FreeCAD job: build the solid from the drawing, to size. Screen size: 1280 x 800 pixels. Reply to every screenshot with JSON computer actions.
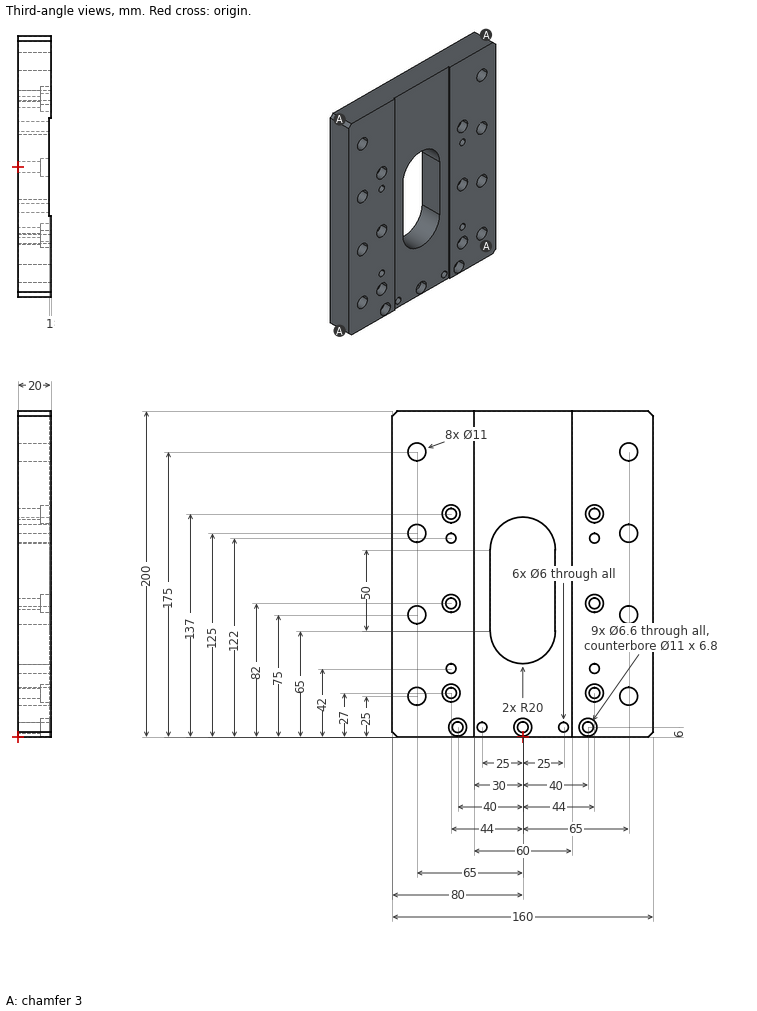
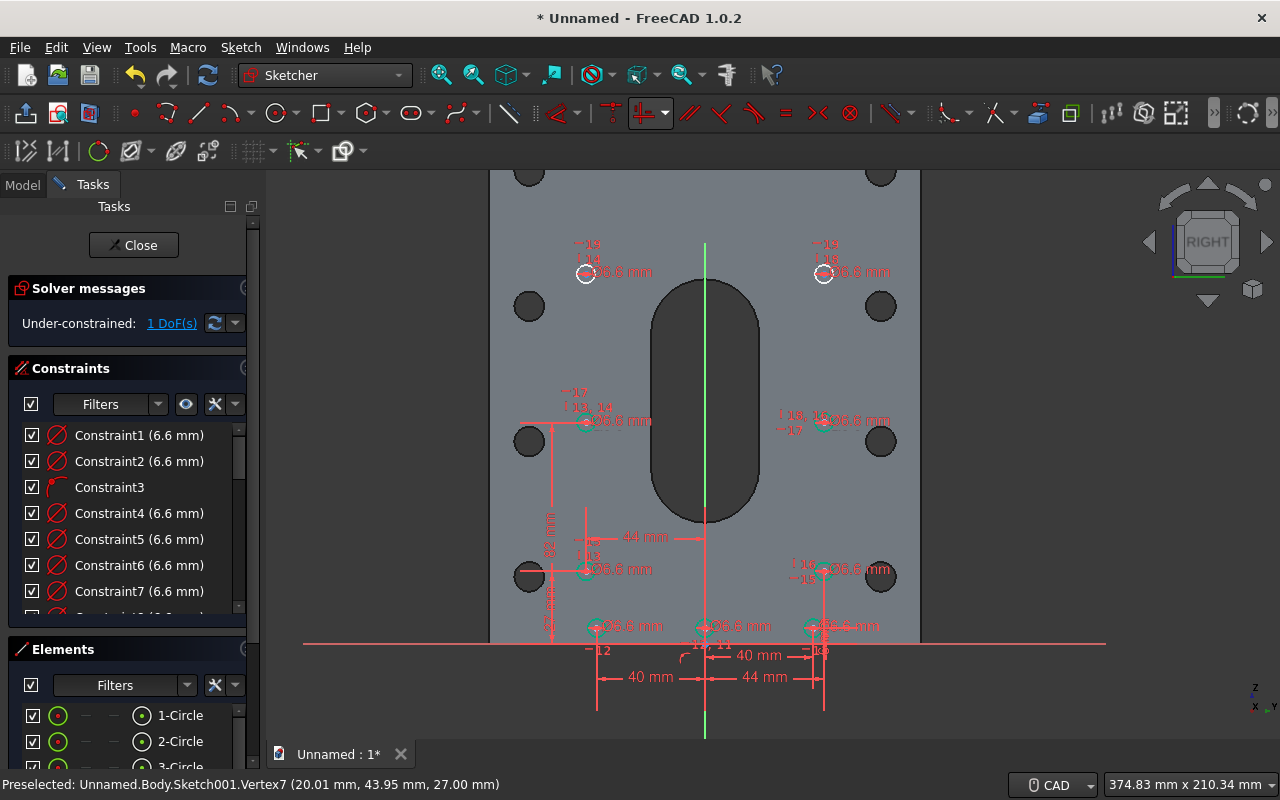
{"action": "left_click", "coordinate": [586, 274]}
{"action": "left_click", "coordinate": [552, 459]}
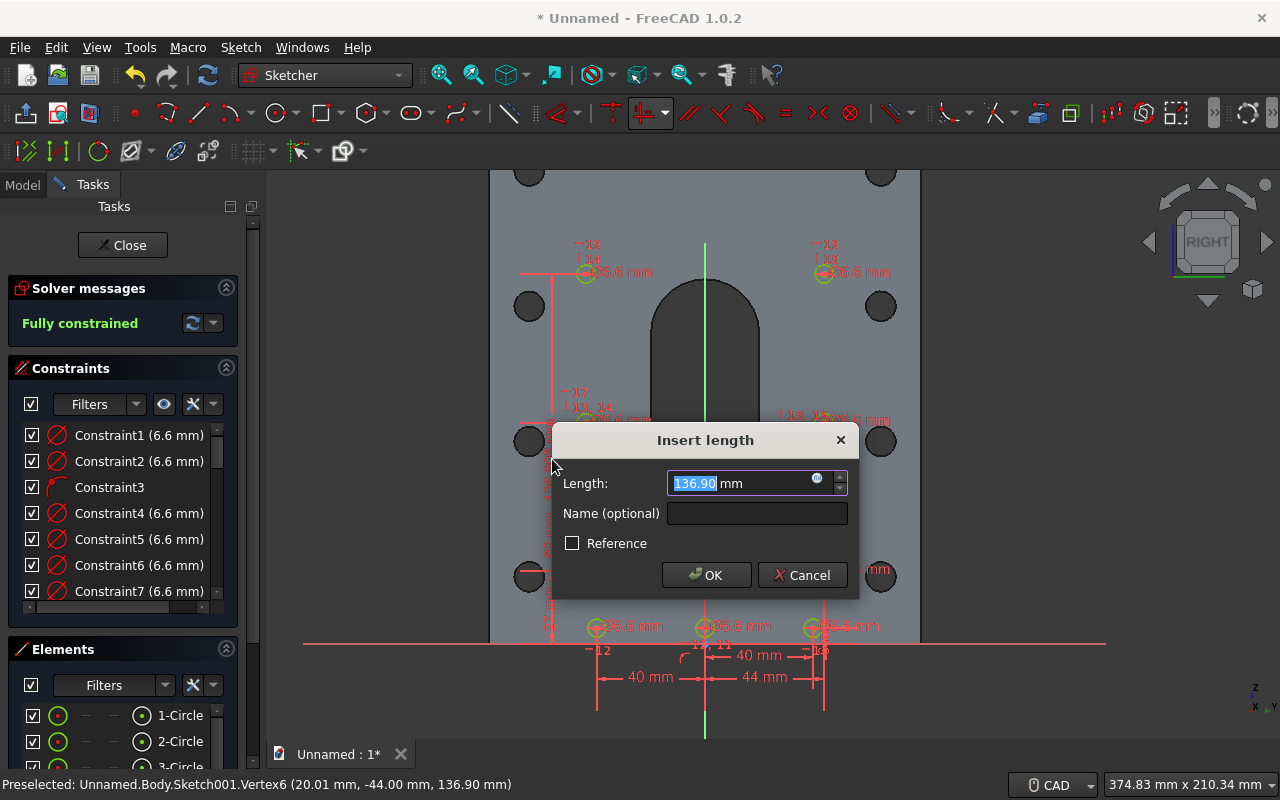
{"action": "type", "text": "137"}
{"action": "key", "text": "Return"}
{"action": "key", "text": "Escape"}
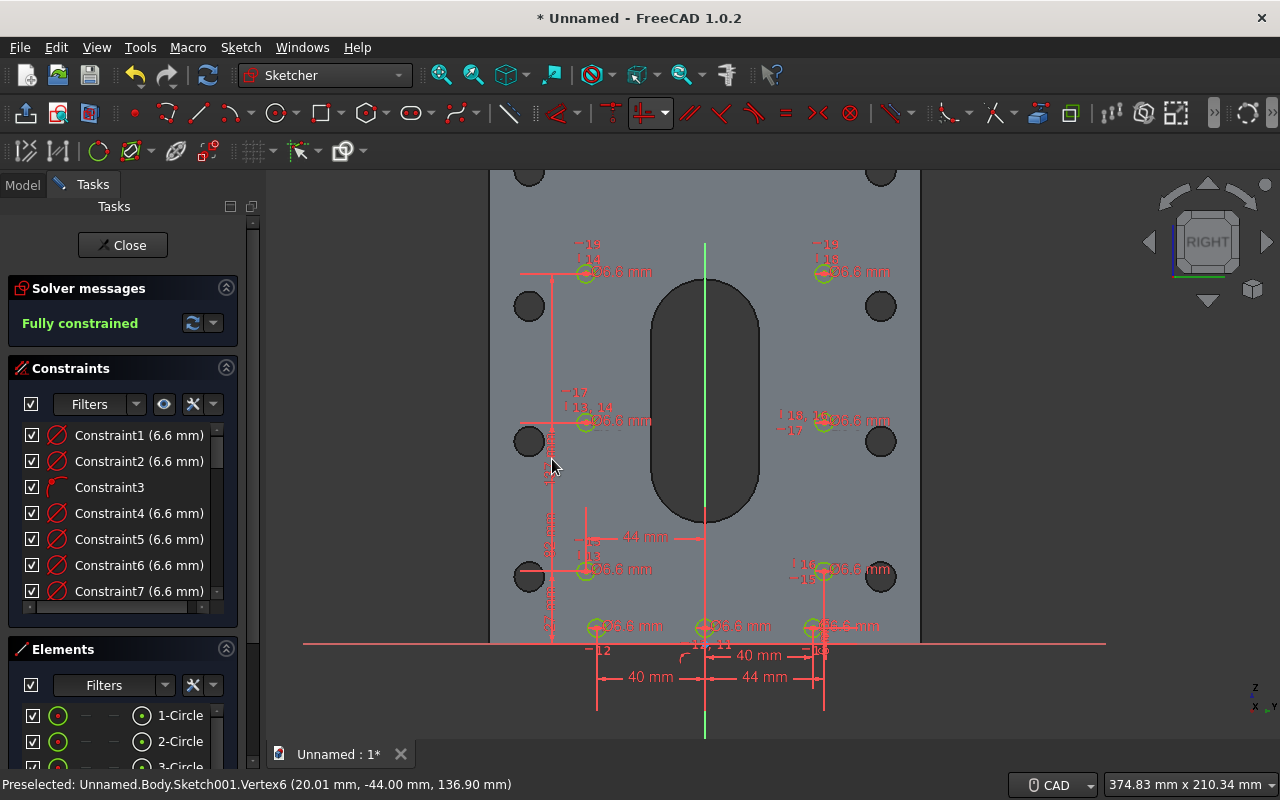
{"action": "left_click", "coordinate": [123, 245]}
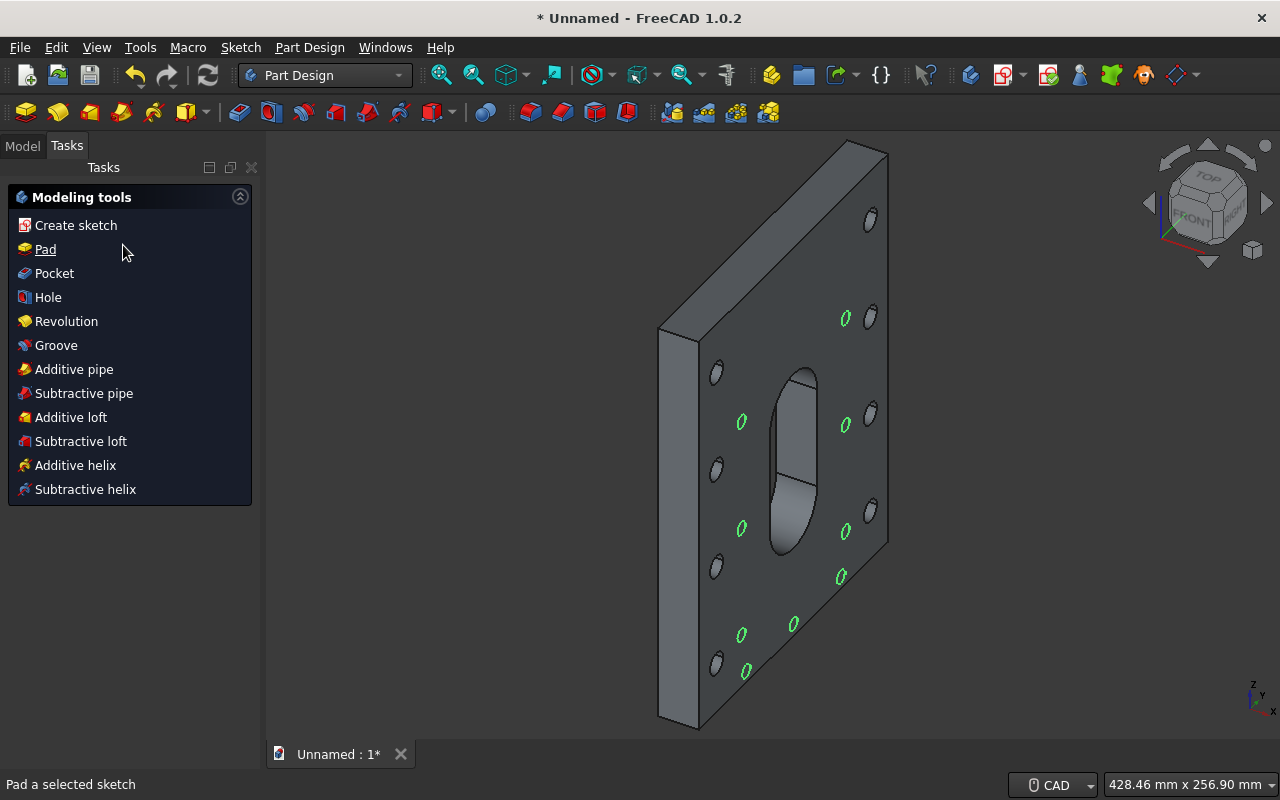
{"action": "left_click", "coordinate": [272, 112]}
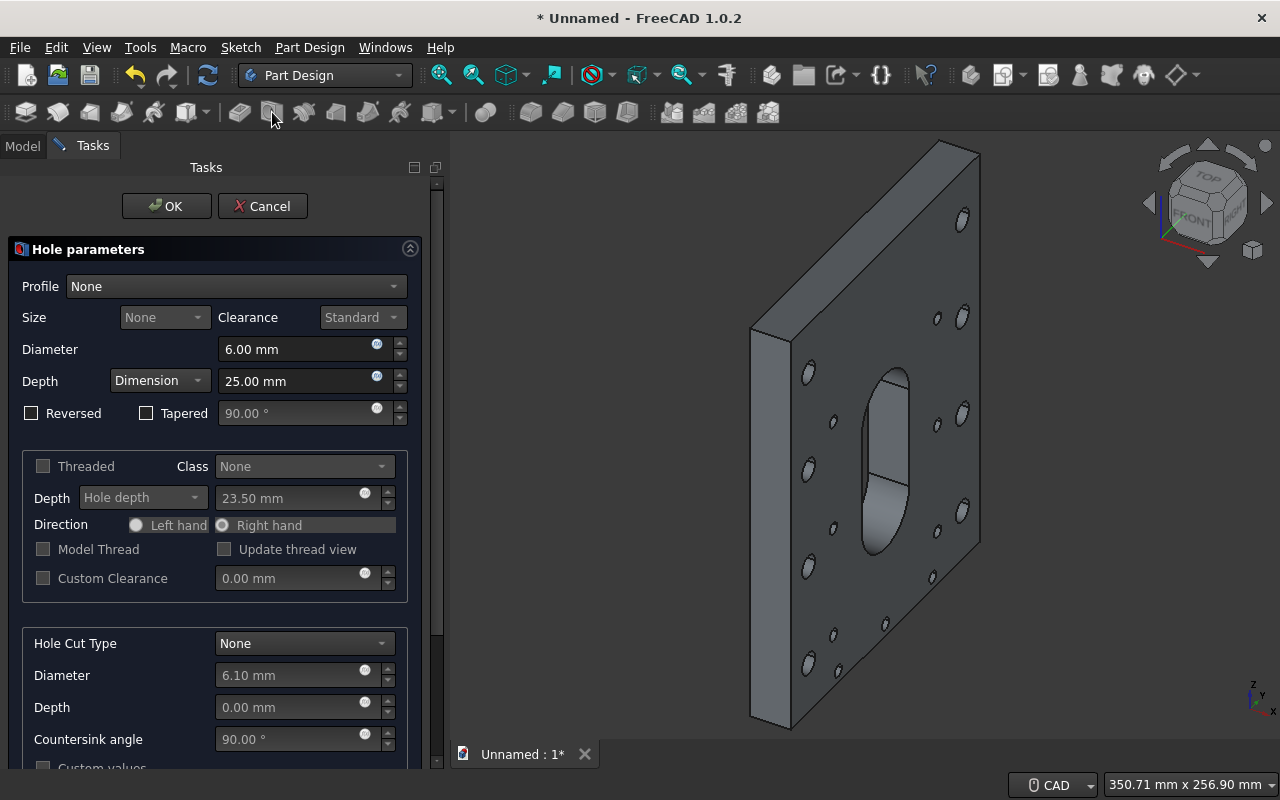
{"action": "triple_click", "coordinate": [305, 349]}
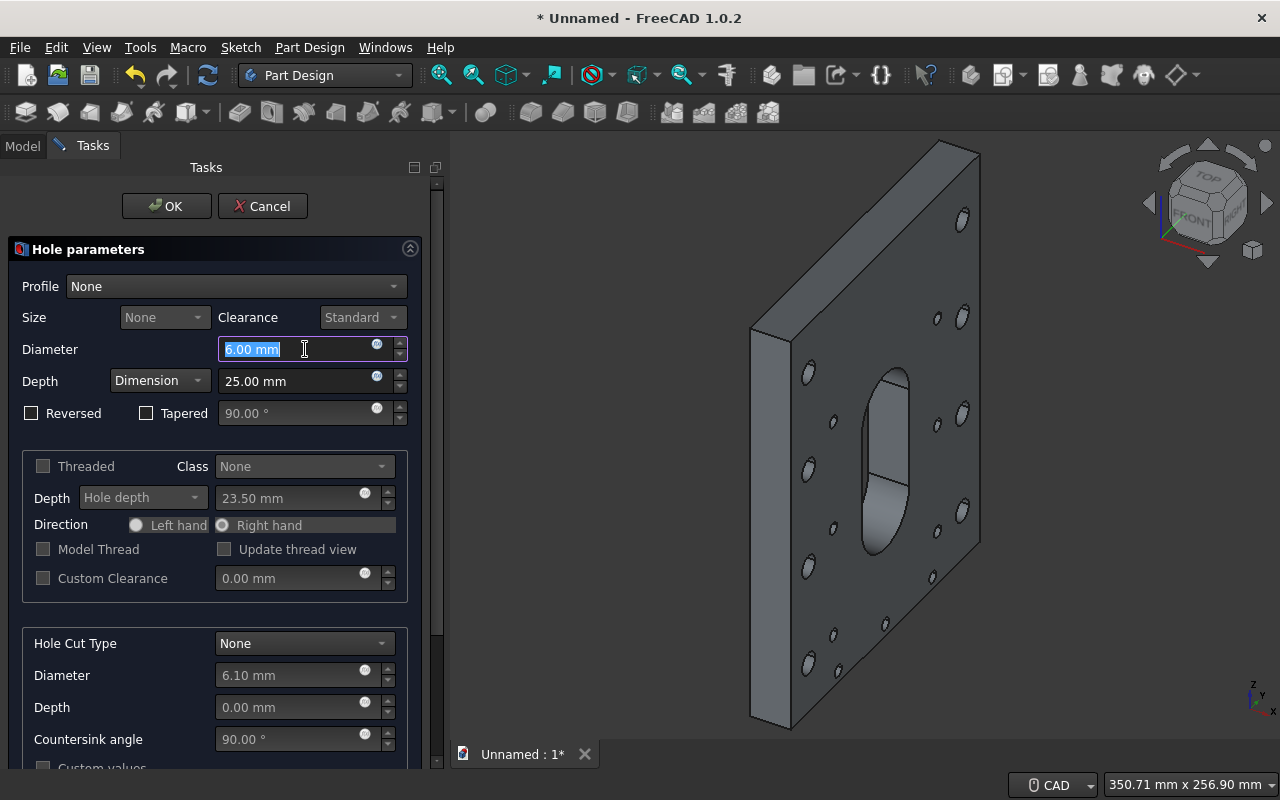
{"action": "type", "text": "6.6"}
{"action": "key", "text": "Tab"}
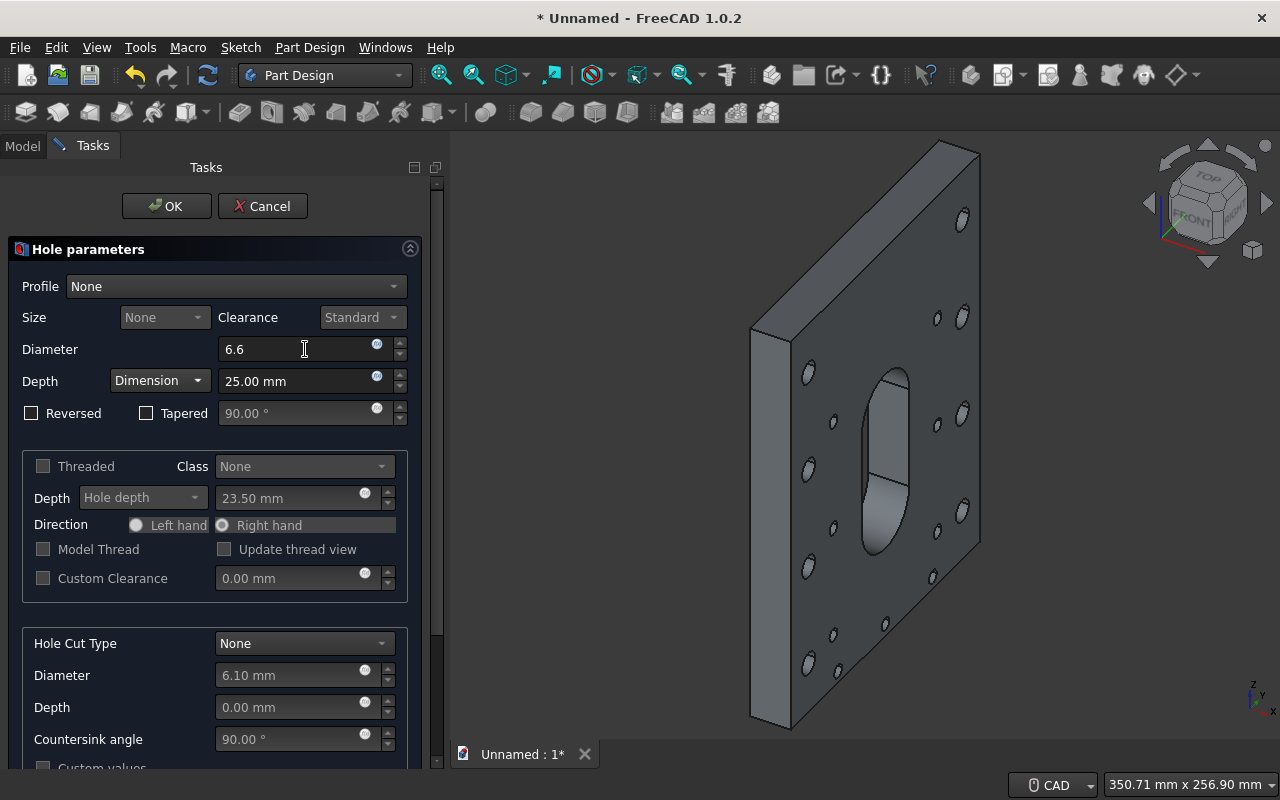
{"action": "left_click", "coordinate": [161, 380]}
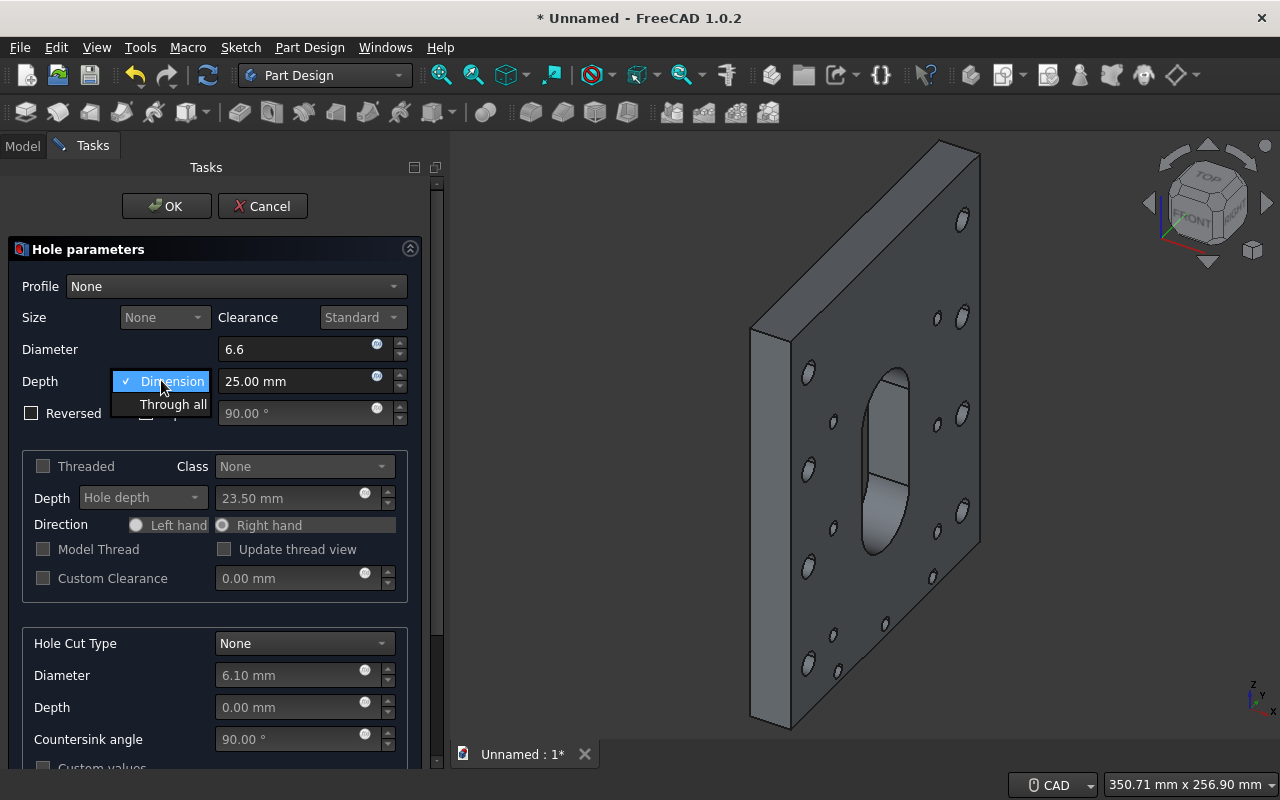
{"action": "left_click", "coordinate": [160, 404]}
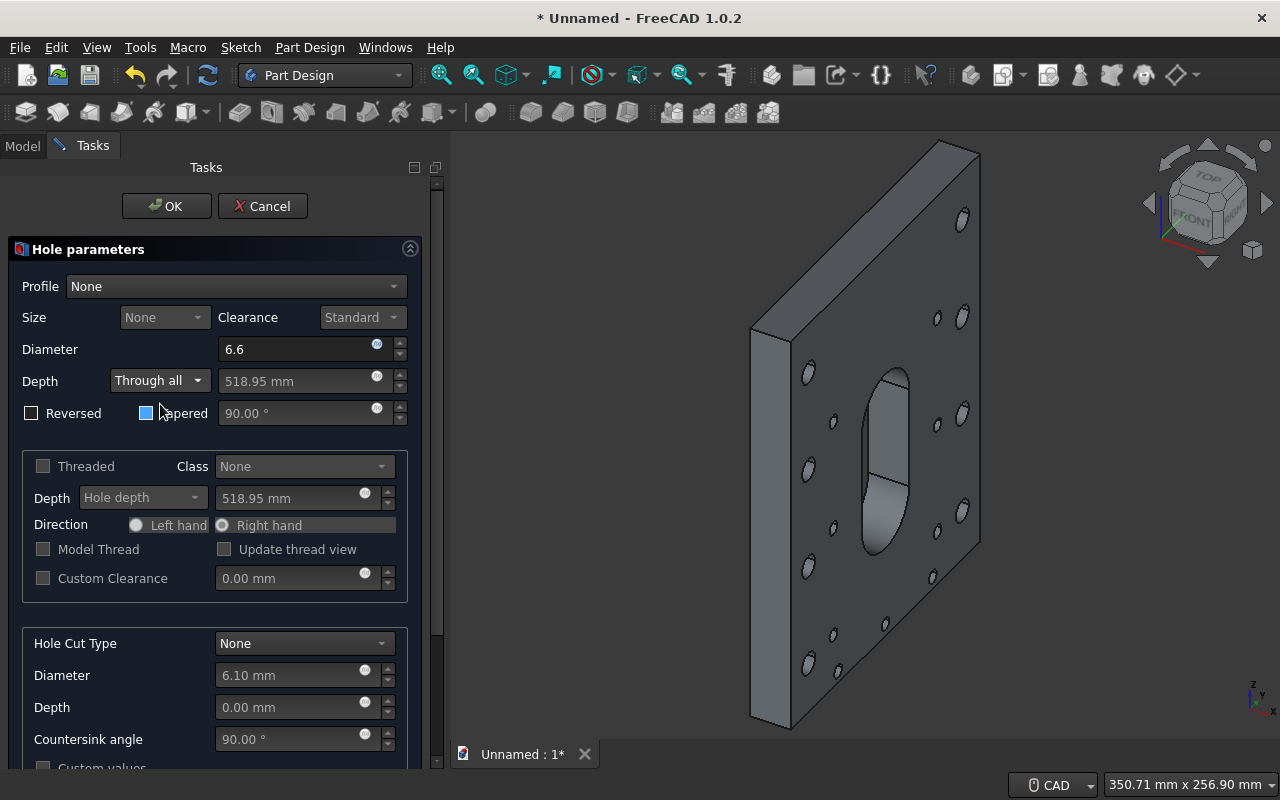
{"action": "left_click", "coordinate": [306, 644]}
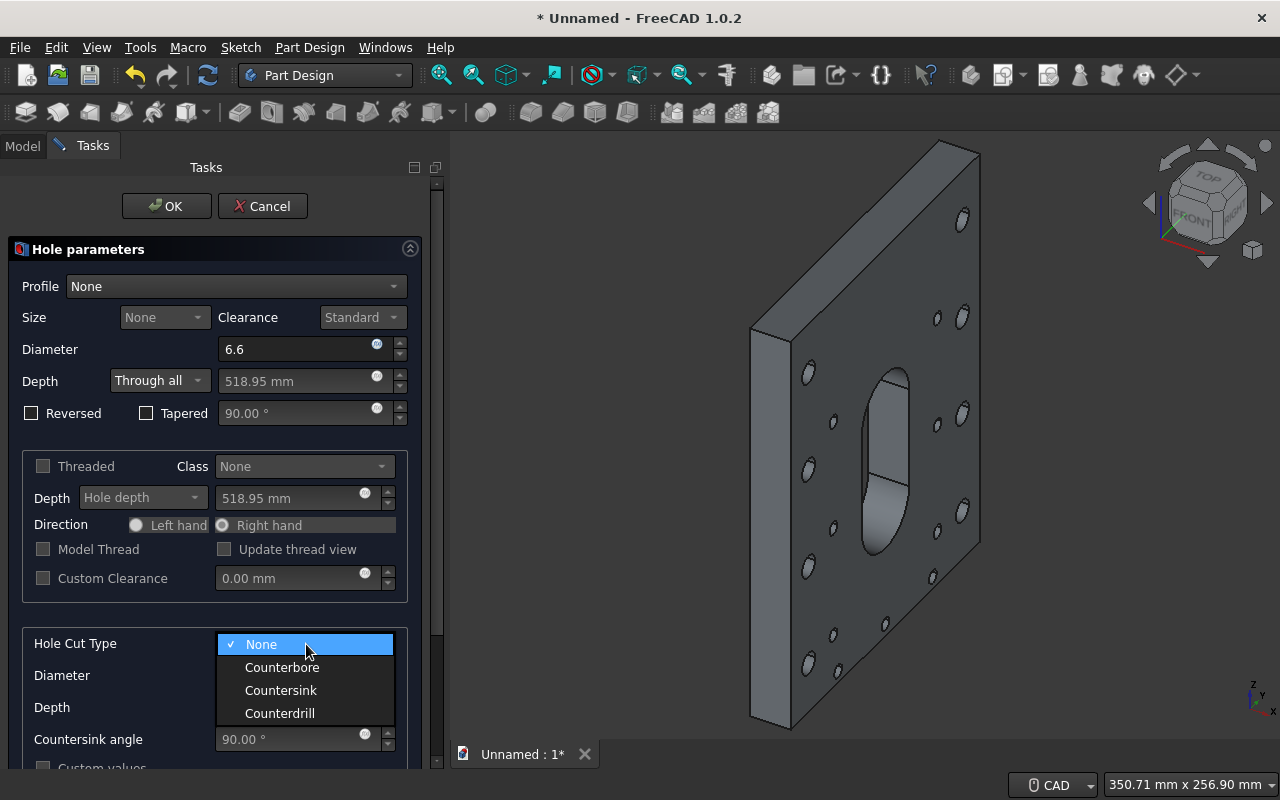
{"action": "left_click", "coordinate": [304, 668]}